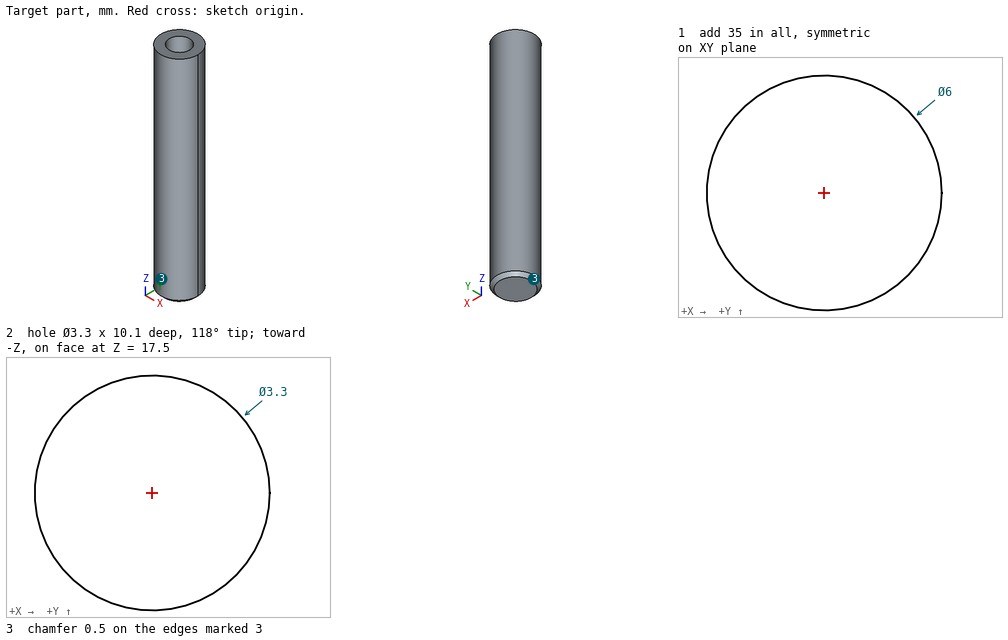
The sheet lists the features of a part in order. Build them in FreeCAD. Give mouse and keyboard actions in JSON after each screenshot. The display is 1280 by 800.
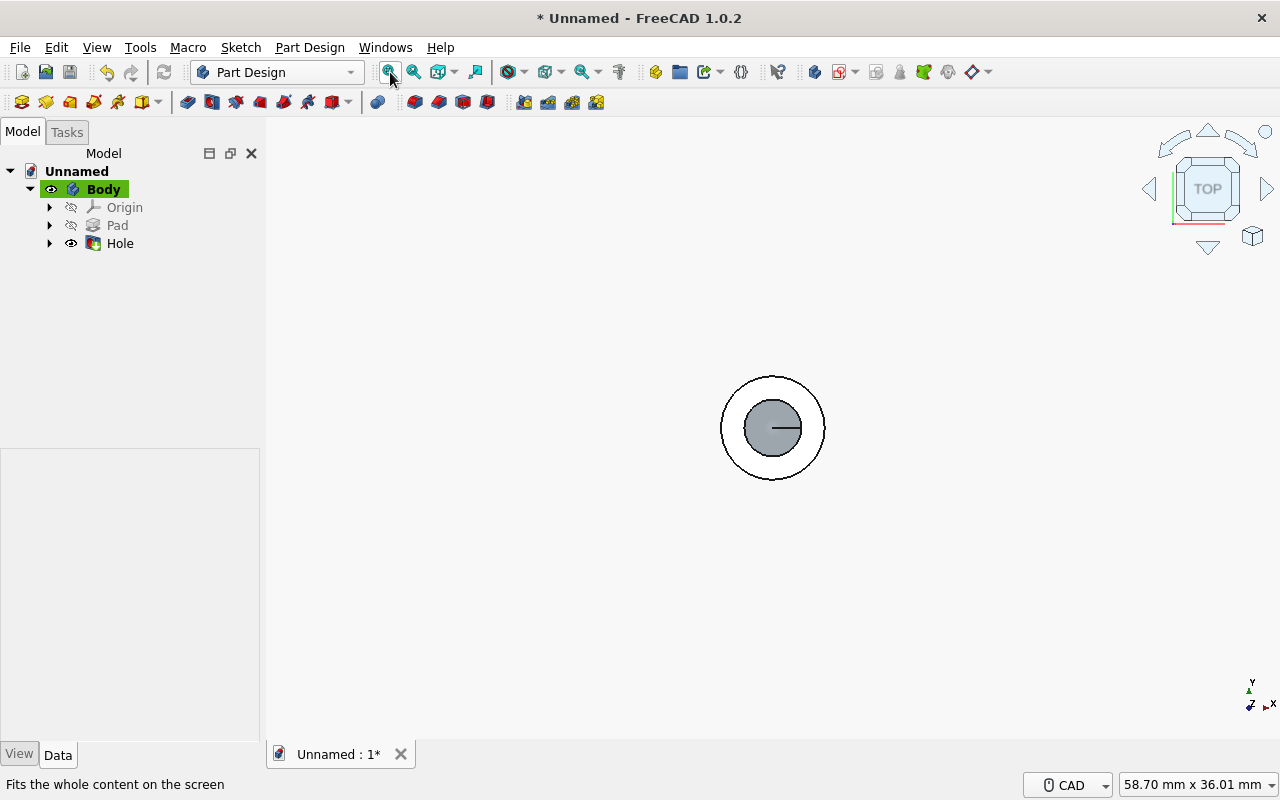
{"action": "key", "text": "1"}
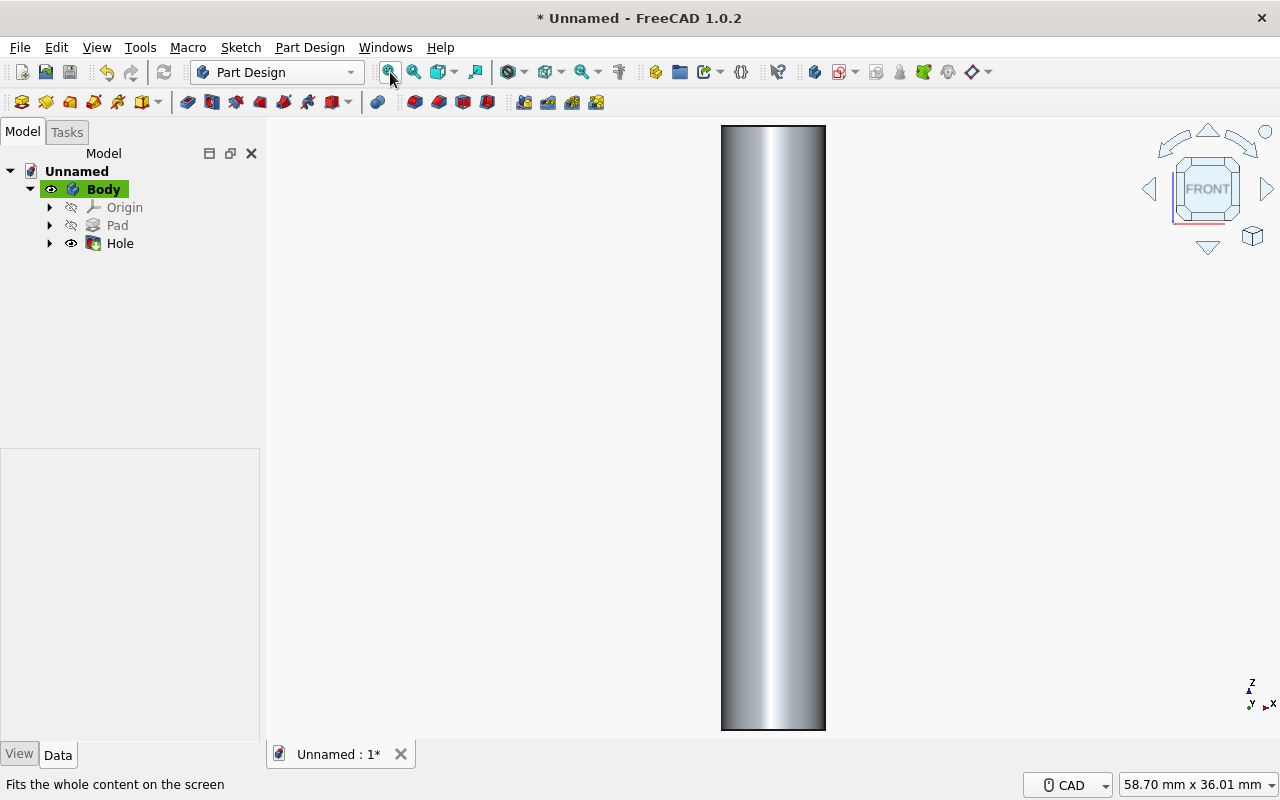
{"action": "key", "text": "3"}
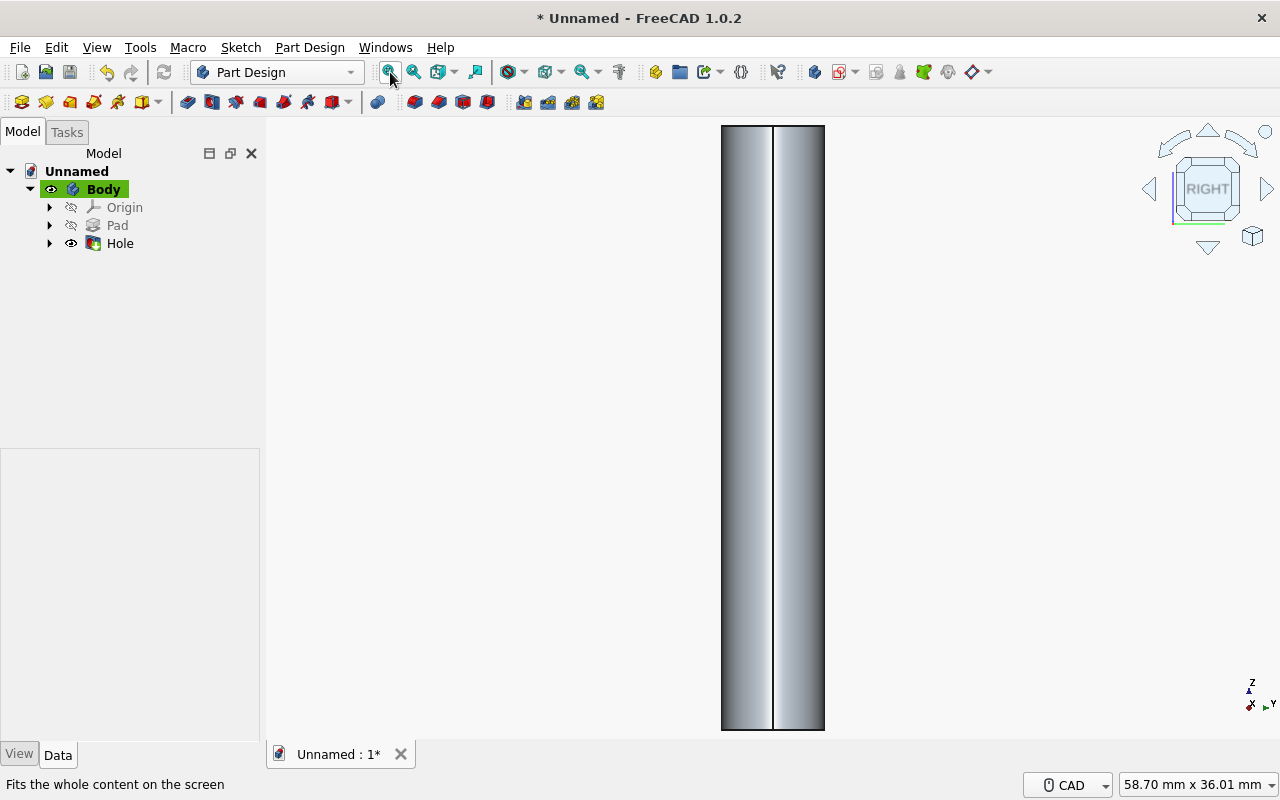
{"action": "key", "text": "5"}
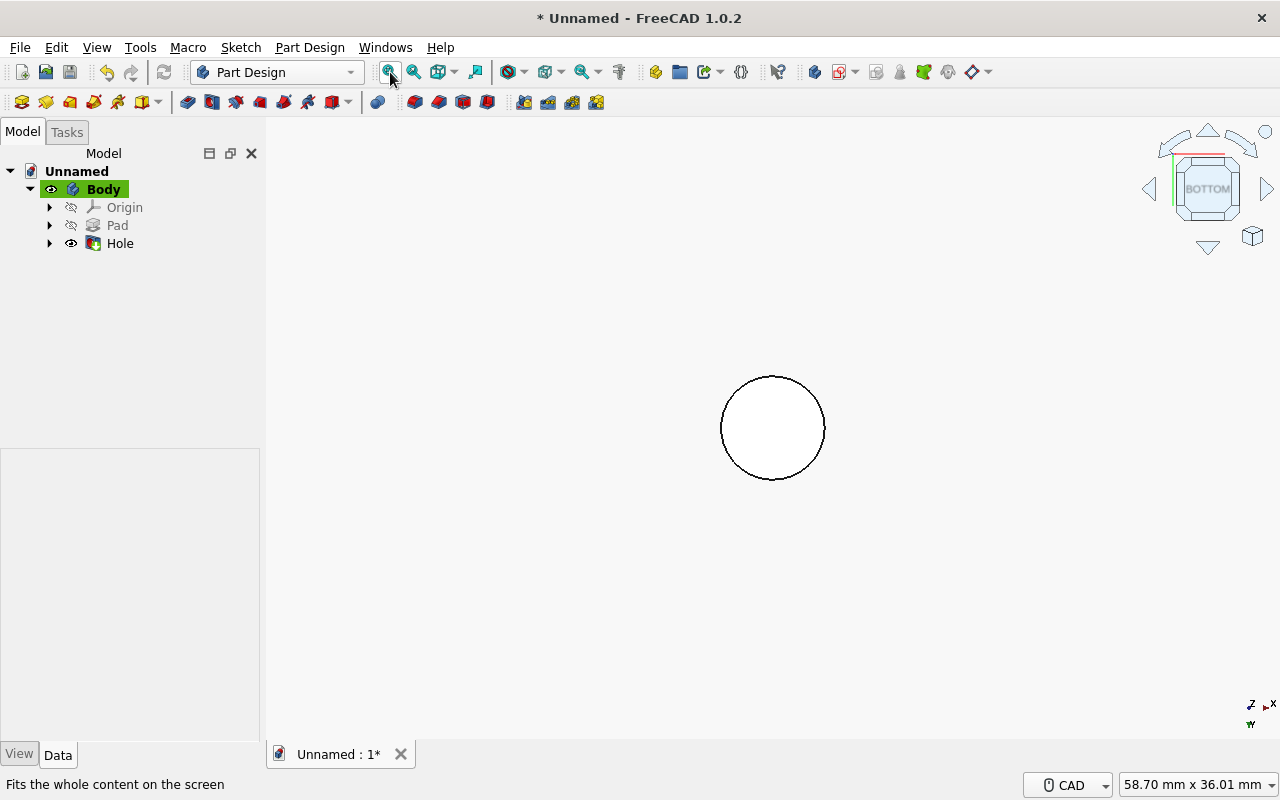
{"action": "left_click", "coordinate": [390, 72]}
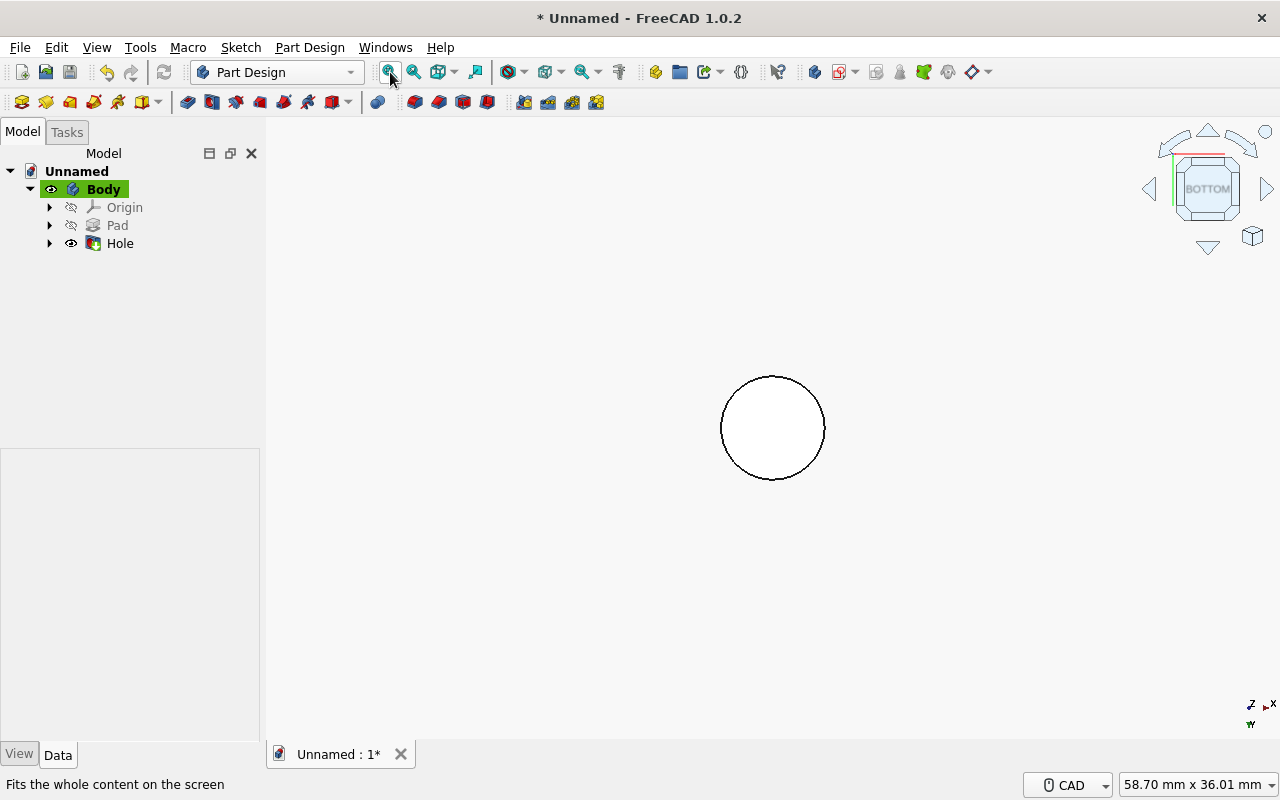
{"action": "left_click", "coordinate": [721, 427]}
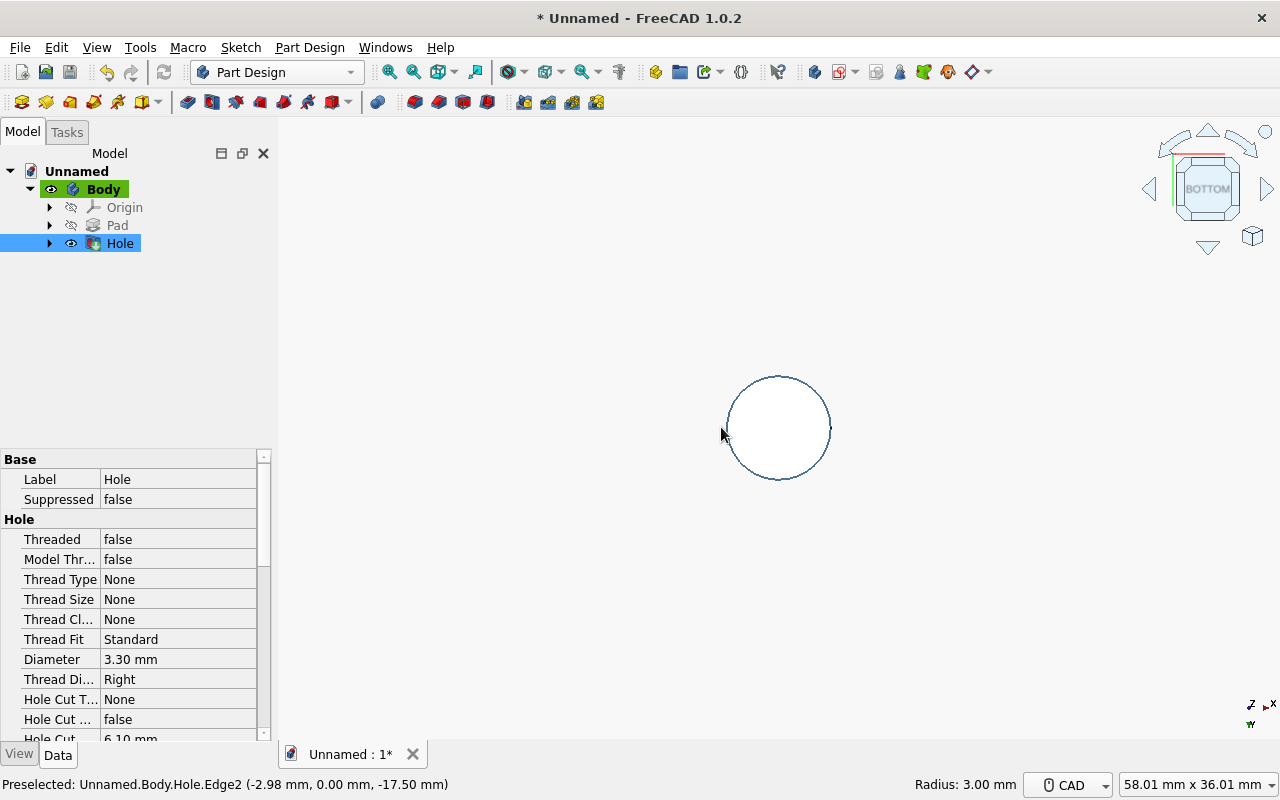
{"action": "left_click", "coordinate": [440, 102]}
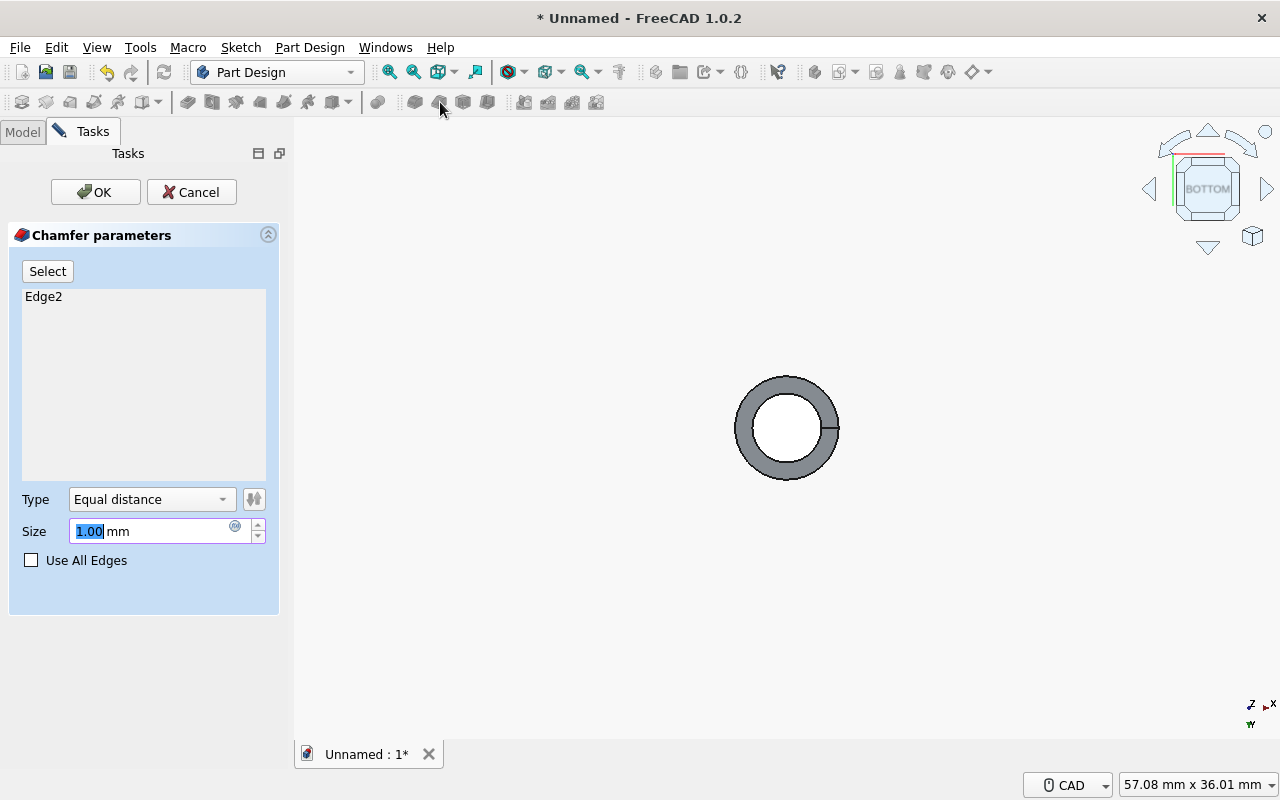
{"action": "type", "text": "0.5"}
{"action": "key", "text": "Tab"}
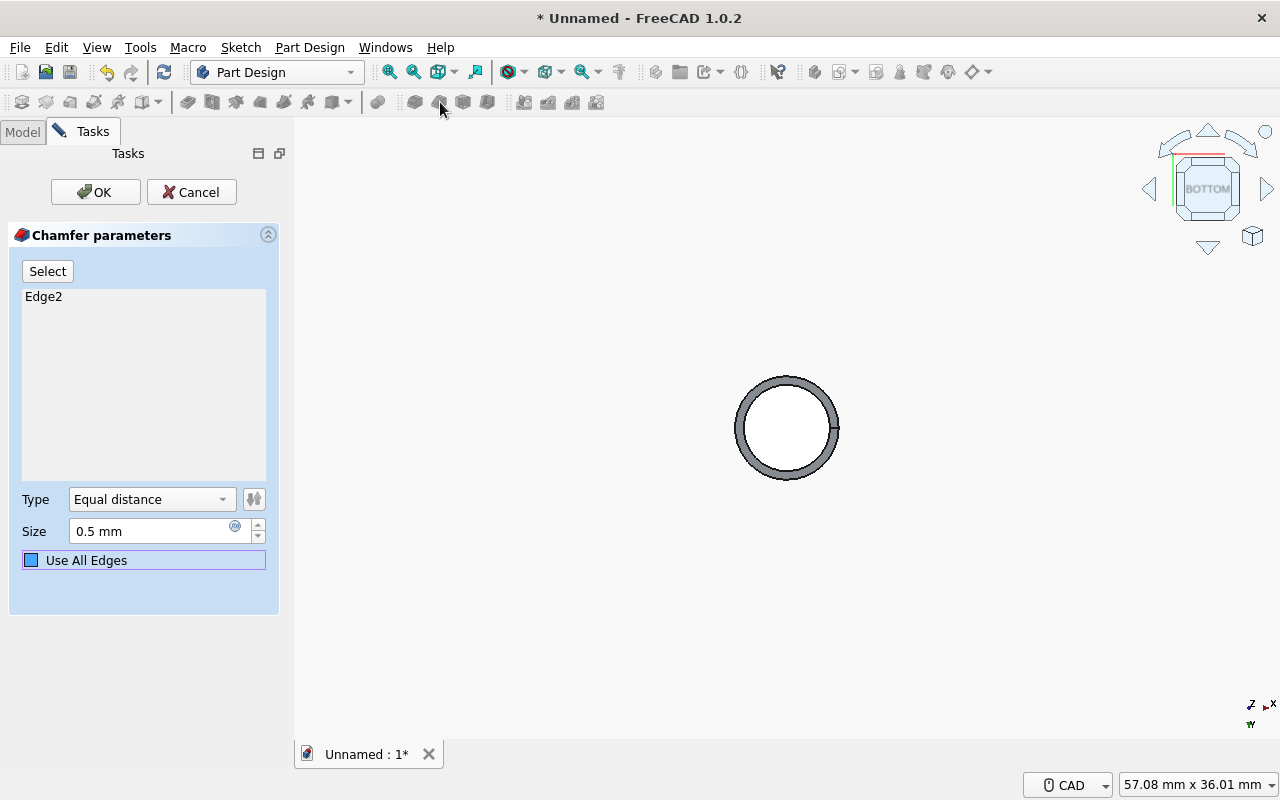
{"action": "left_click", "coordinate": [96, 192]}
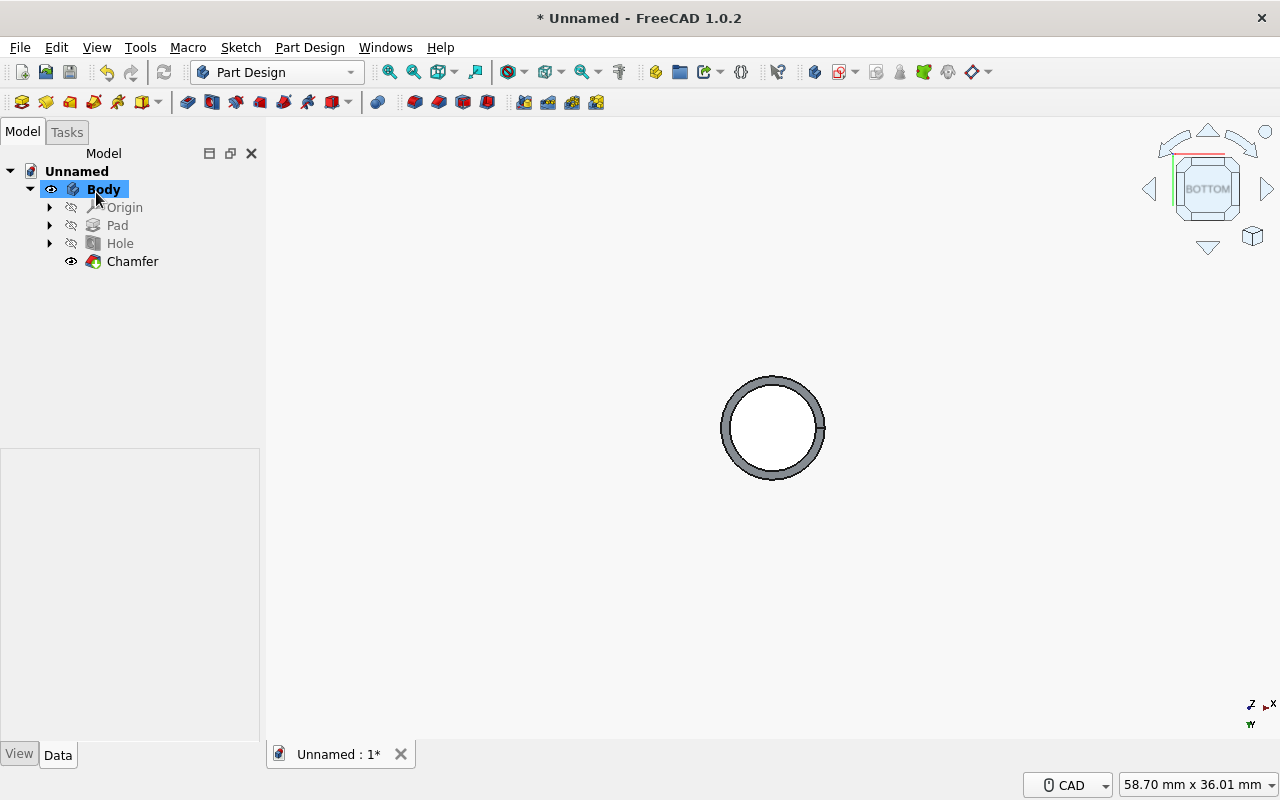
{"action": "key", "text": "0"}